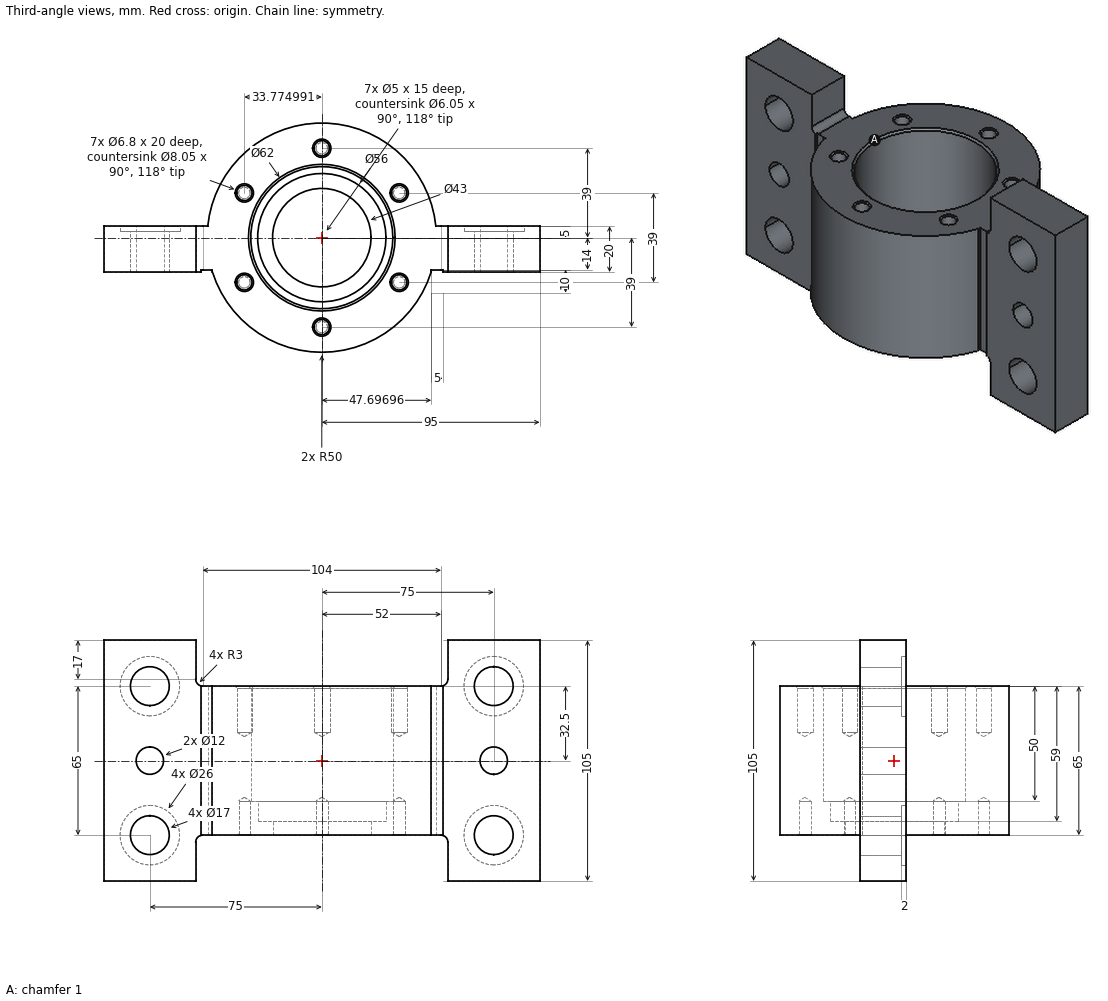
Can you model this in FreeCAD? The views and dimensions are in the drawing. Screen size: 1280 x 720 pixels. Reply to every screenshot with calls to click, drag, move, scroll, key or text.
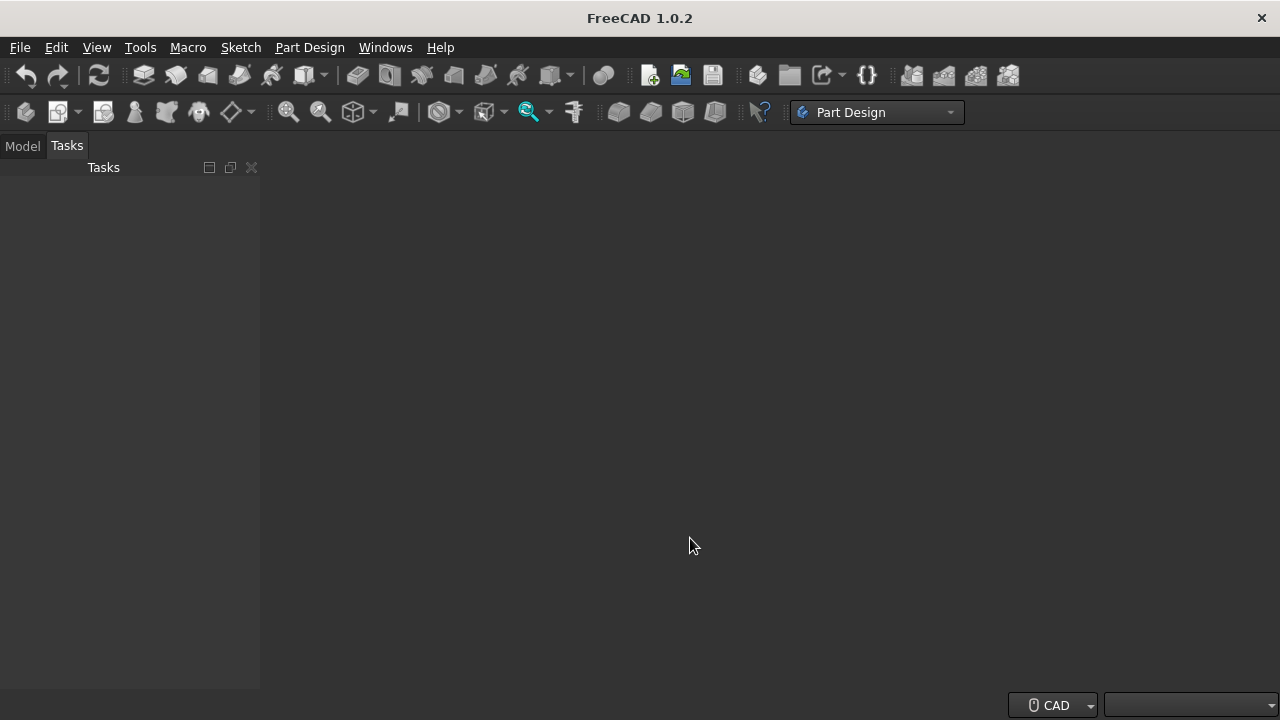
click(650, 76)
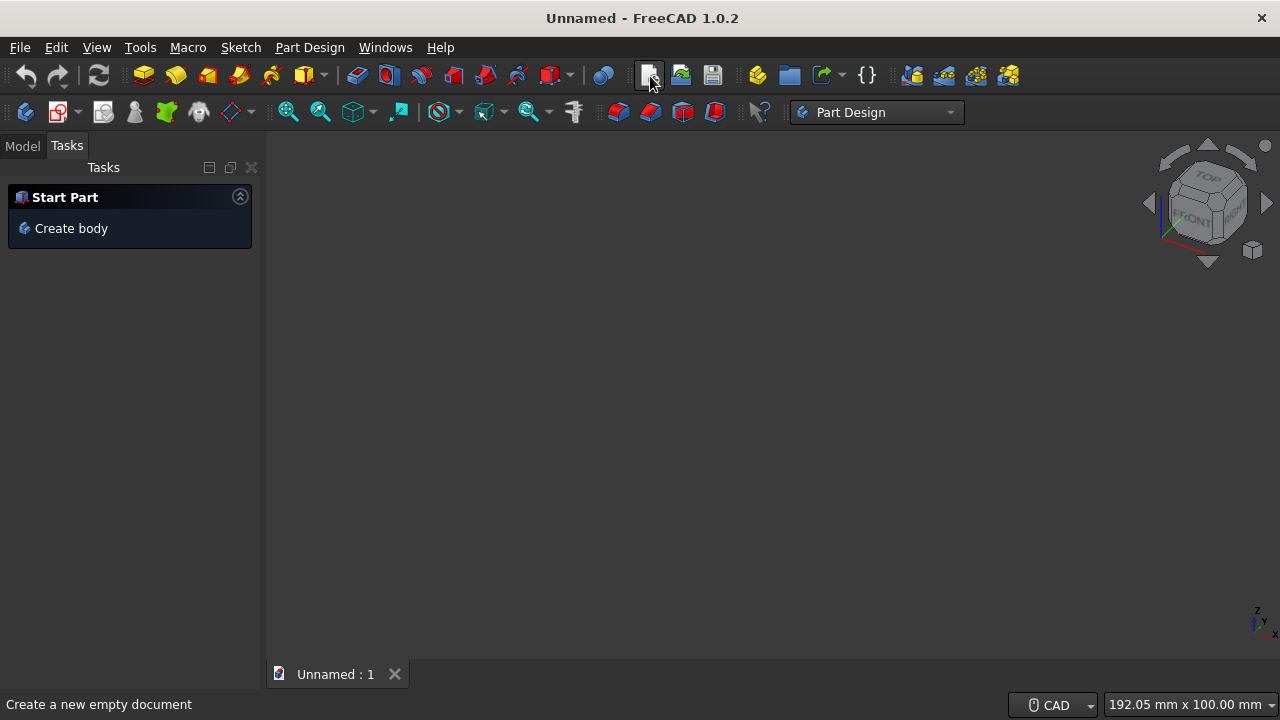
click(58, 112)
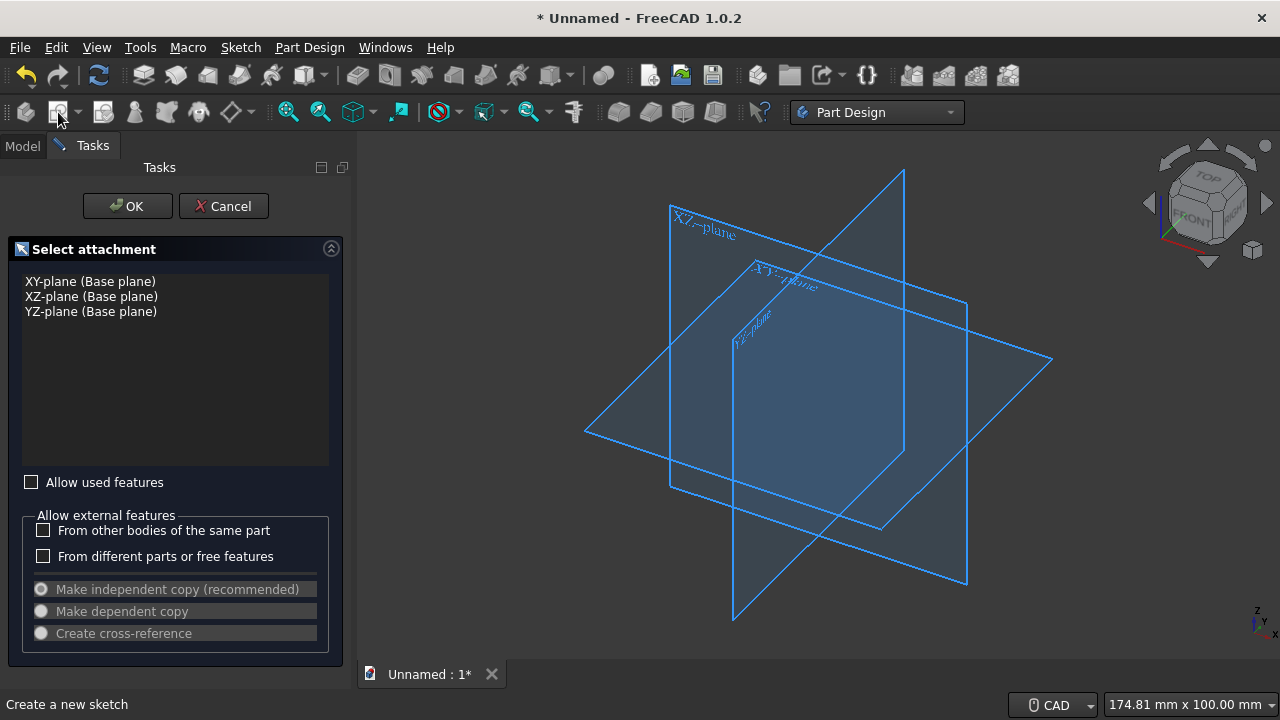
click(82, 282)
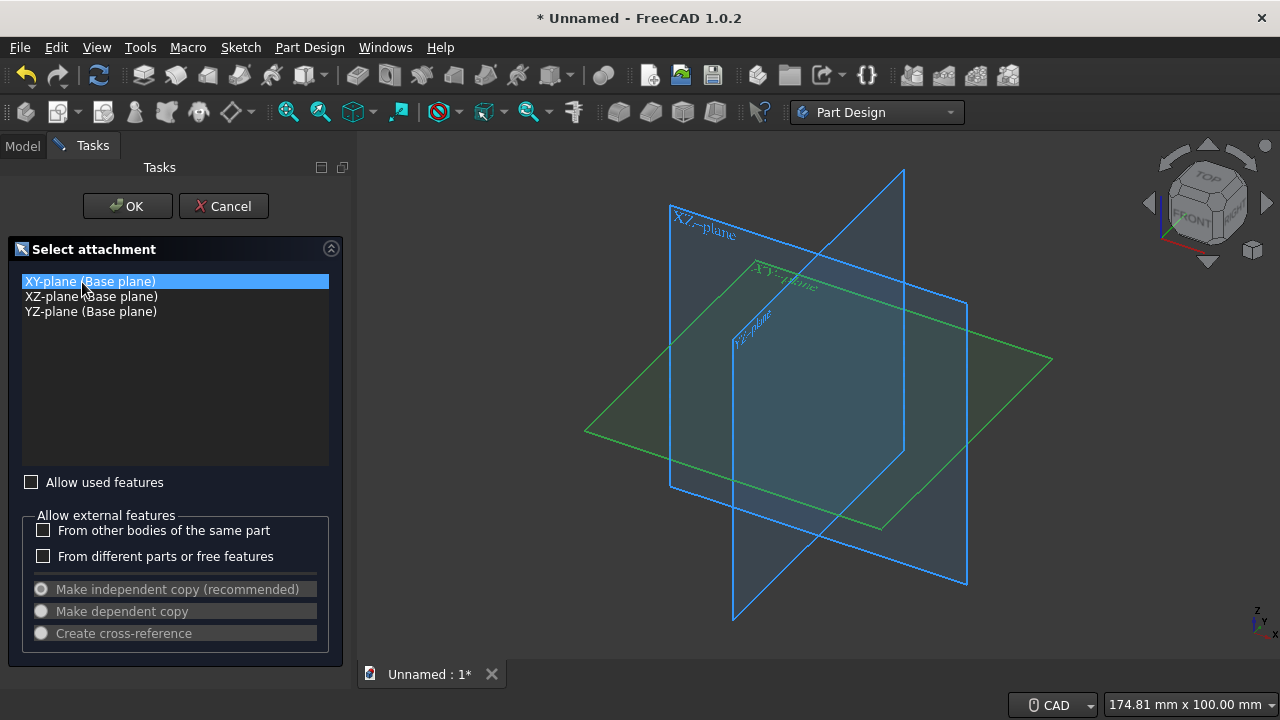
click(128, 206)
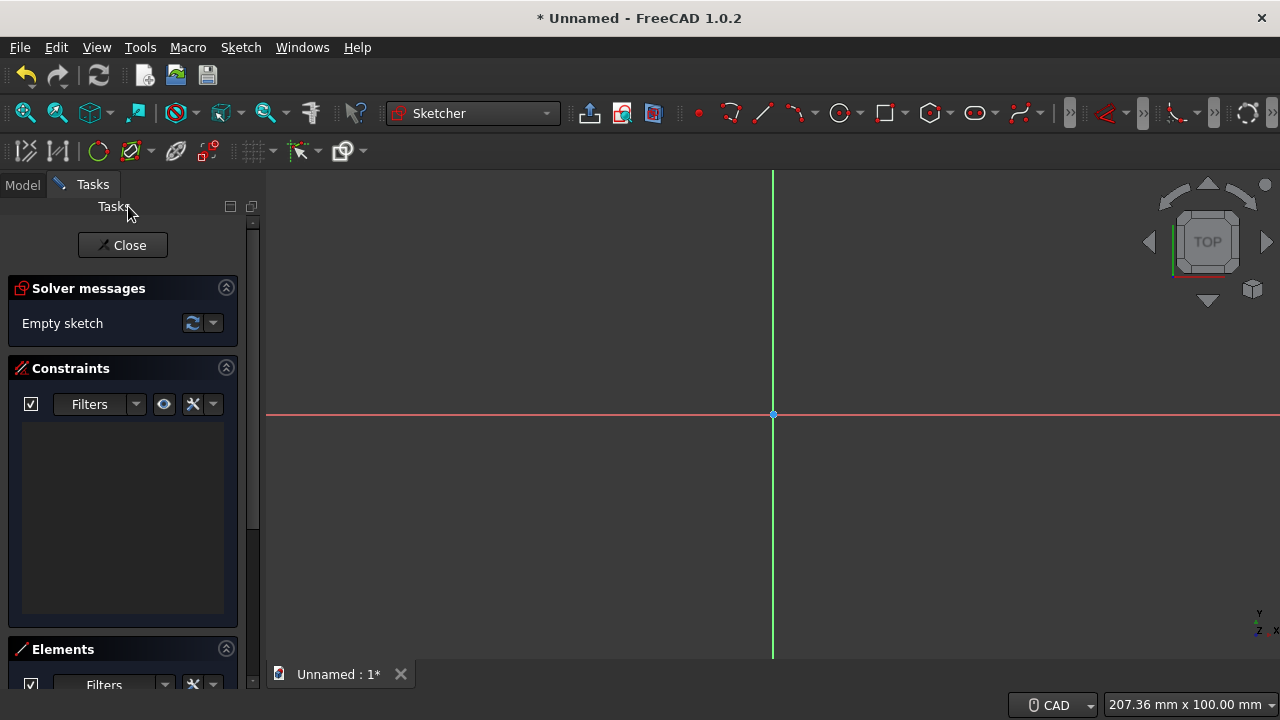
scroll(565, 414, down, 2)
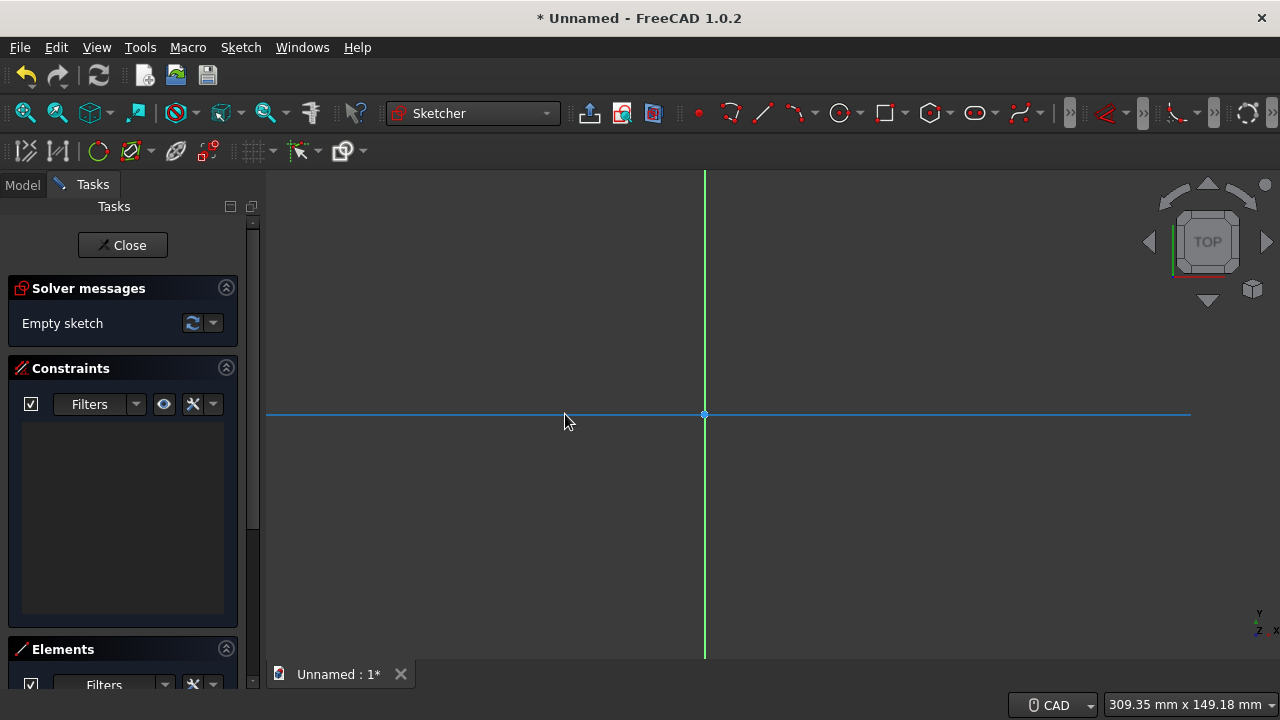
click(732, 114)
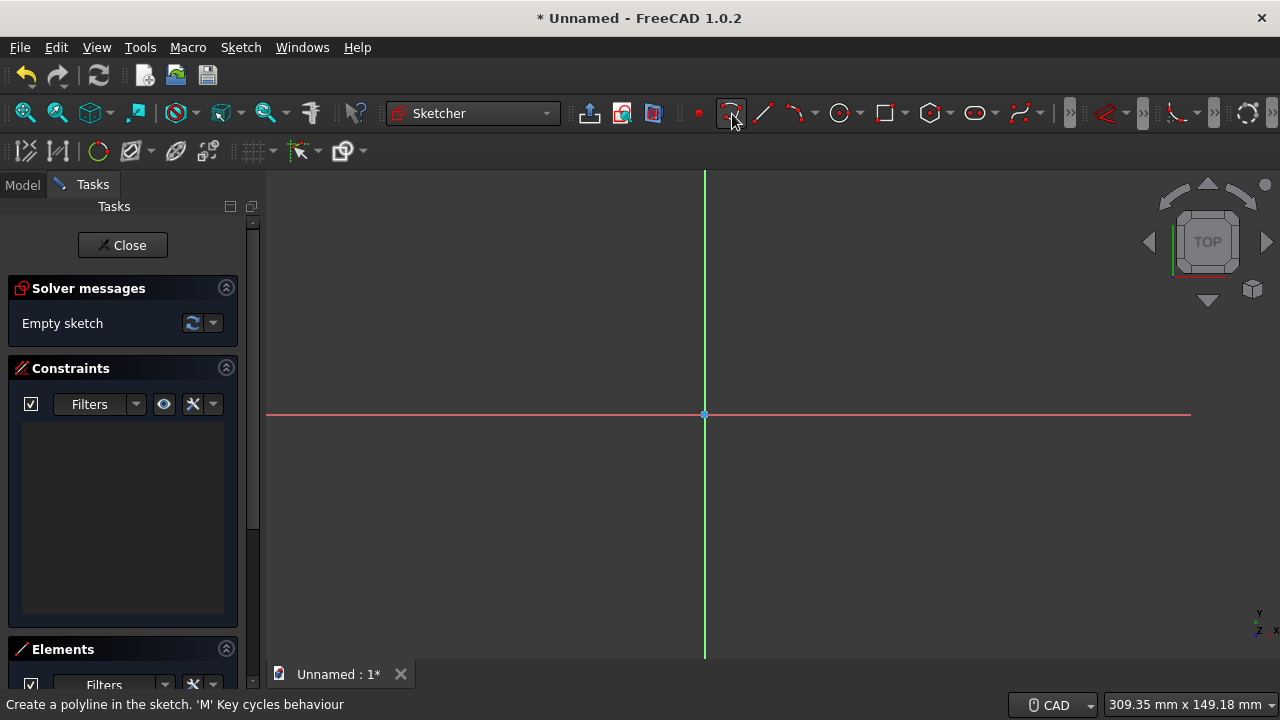
click(861, 464)
click(1016, 464)
click(1016, 398)
click(868, 398)
right_click(868, 398)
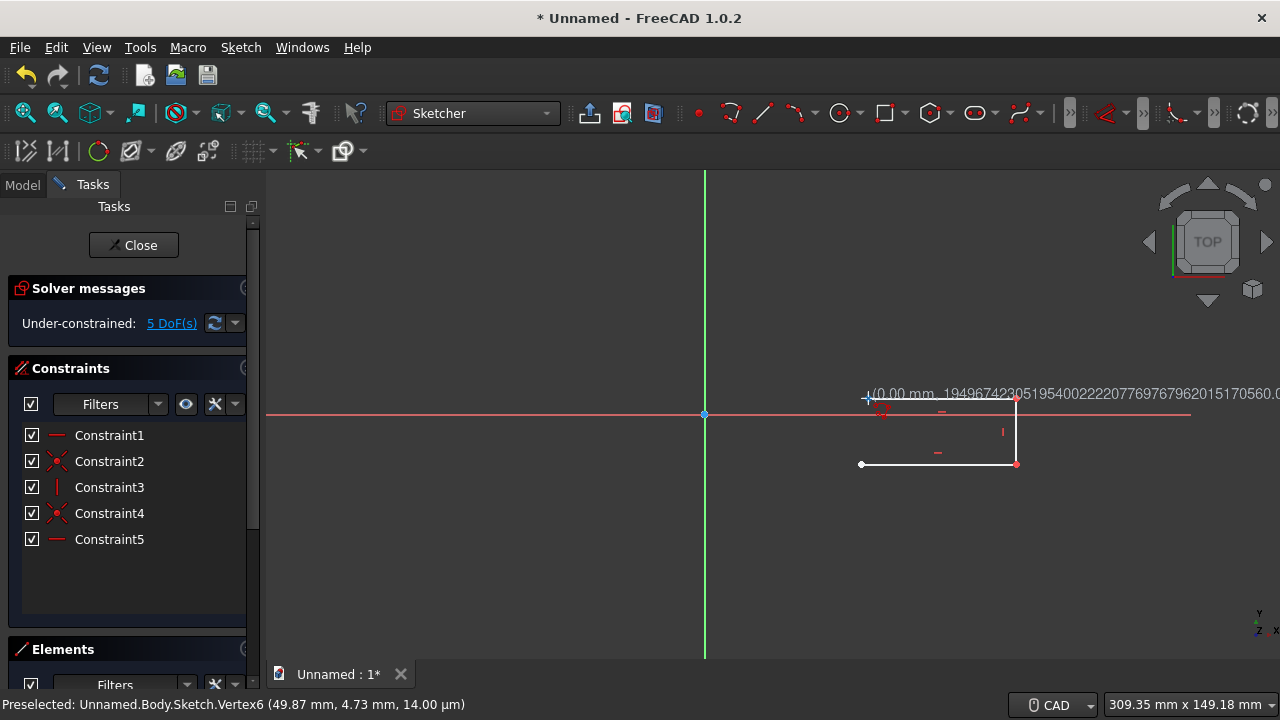
click(541, 398)
click(393, 398)
click(393, 464)
click(548, 464)
right_click(548, 464)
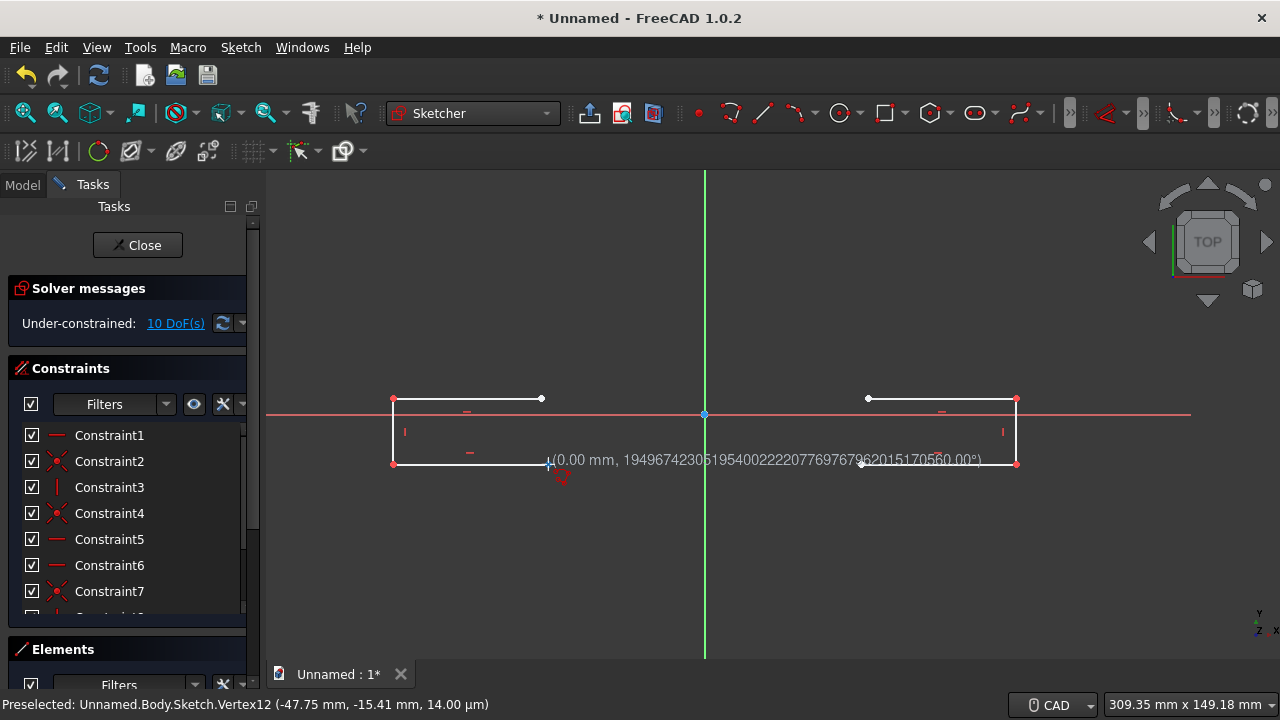
click(796, 114)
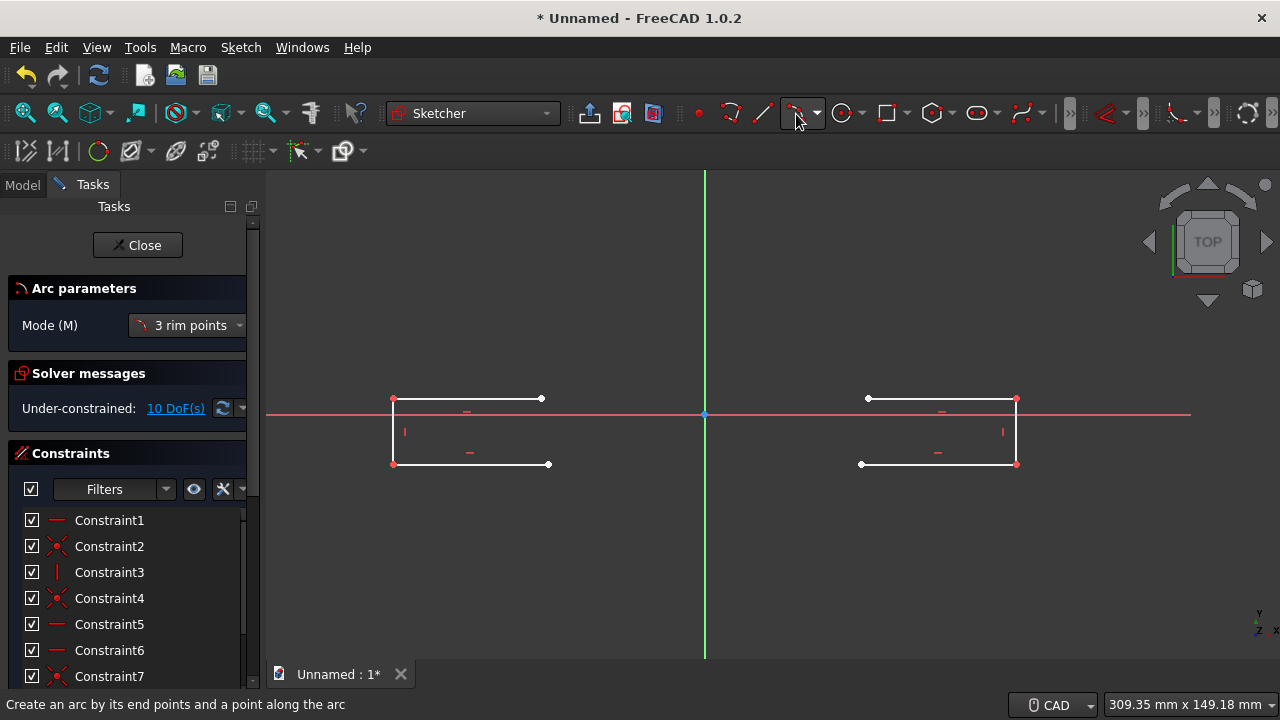
click(868, 399)
click(541, 399)
click(752, 258)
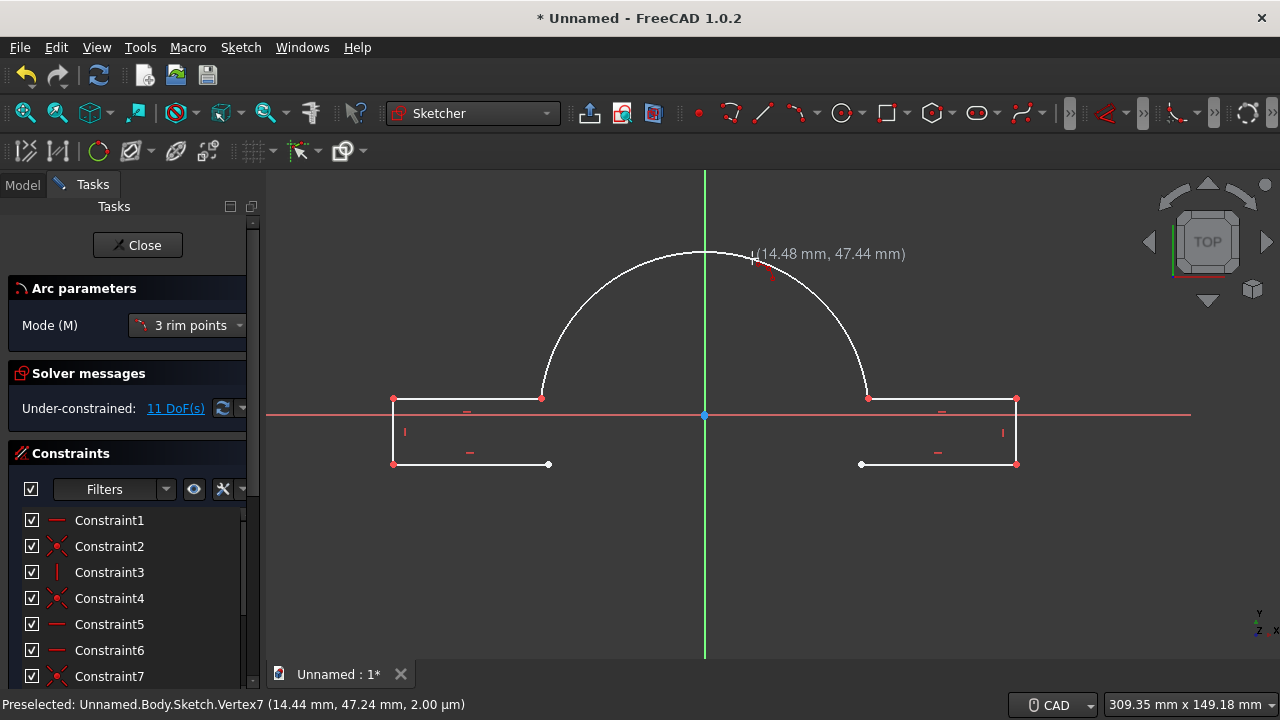
click(548, 465)
click(861, 465)
click(663, 573)
key(Escape)